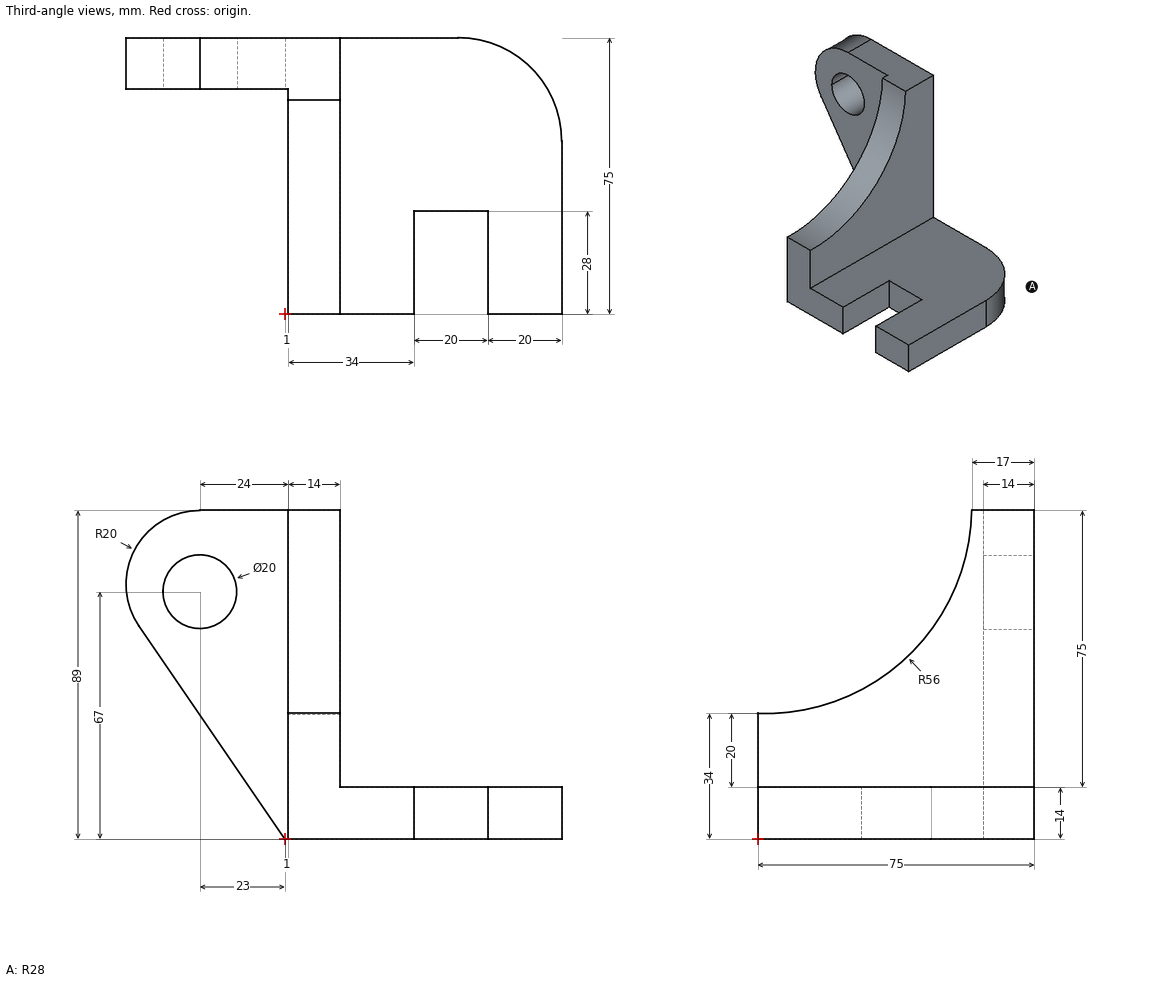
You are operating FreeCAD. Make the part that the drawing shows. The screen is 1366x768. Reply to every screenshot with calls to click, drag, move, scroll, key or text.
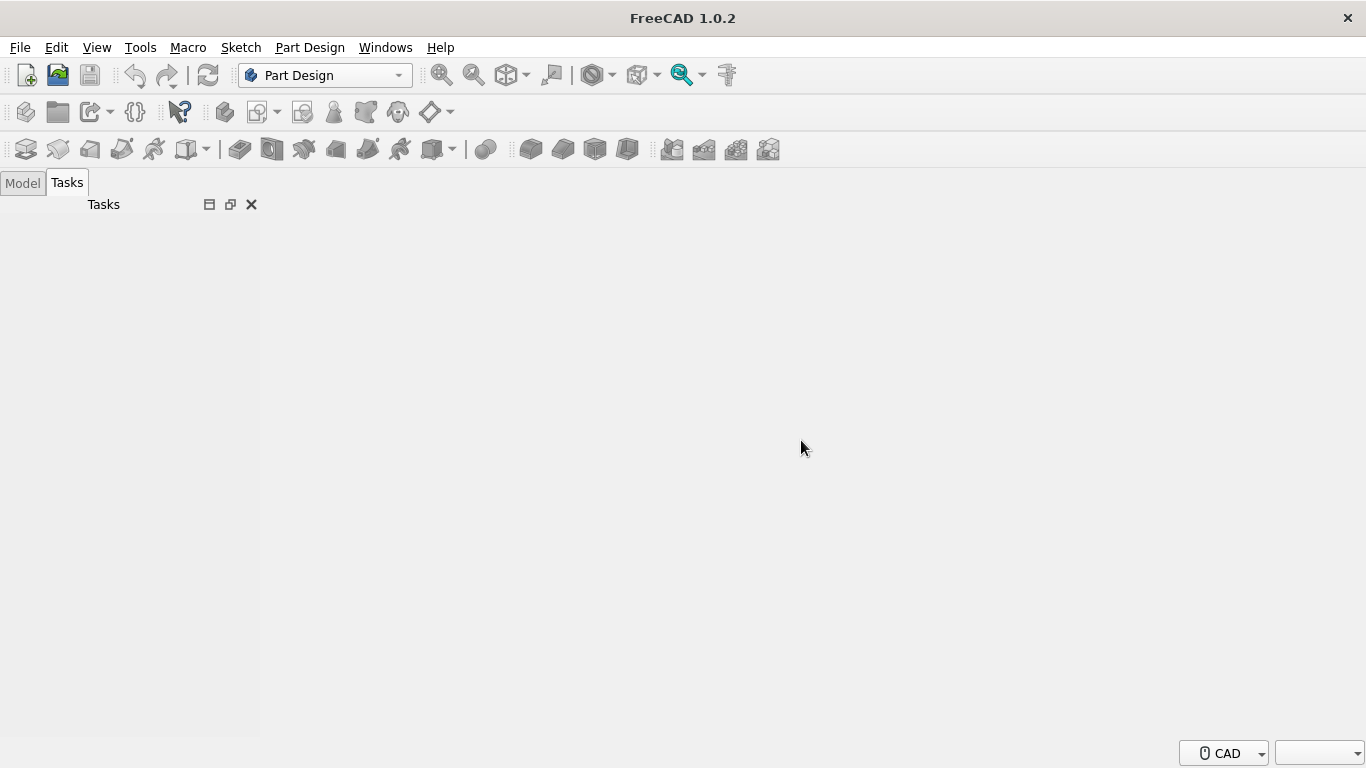
click(26, 76)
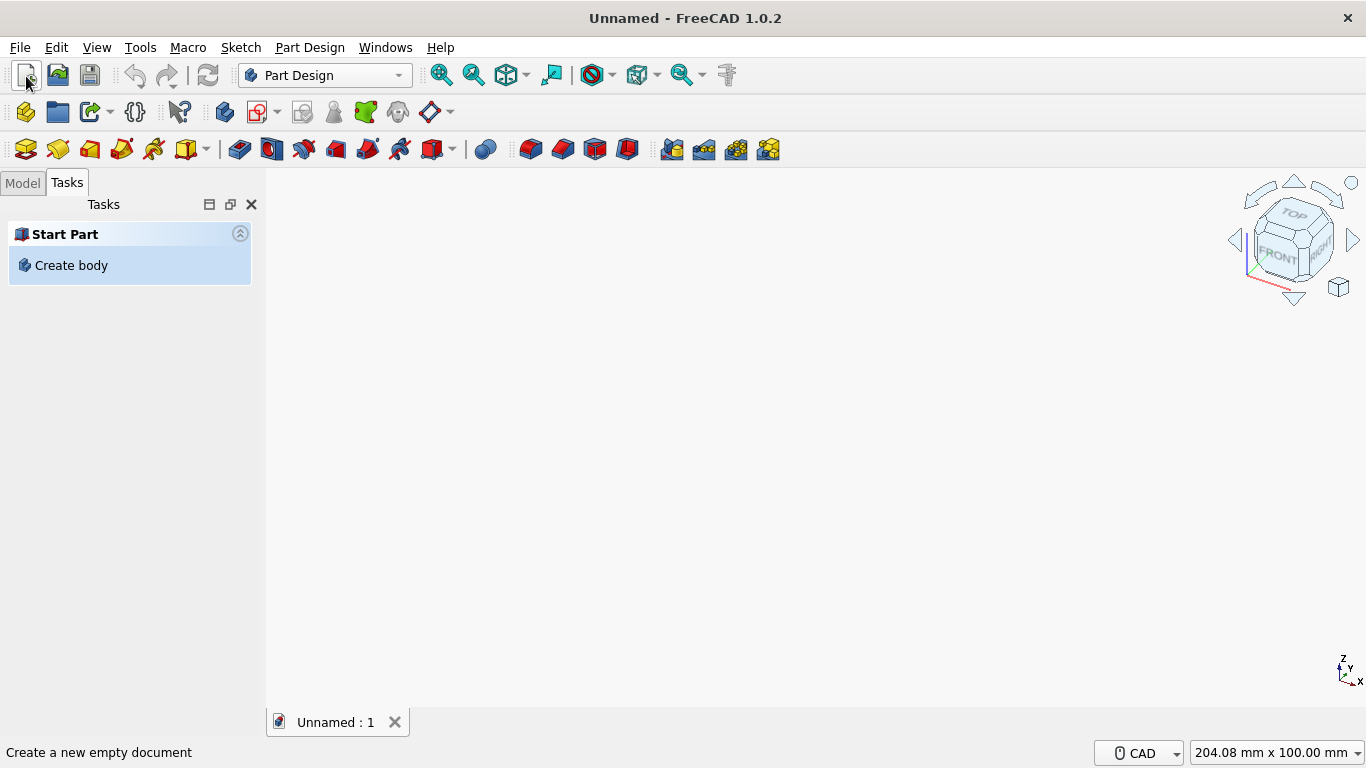
click(258, 112)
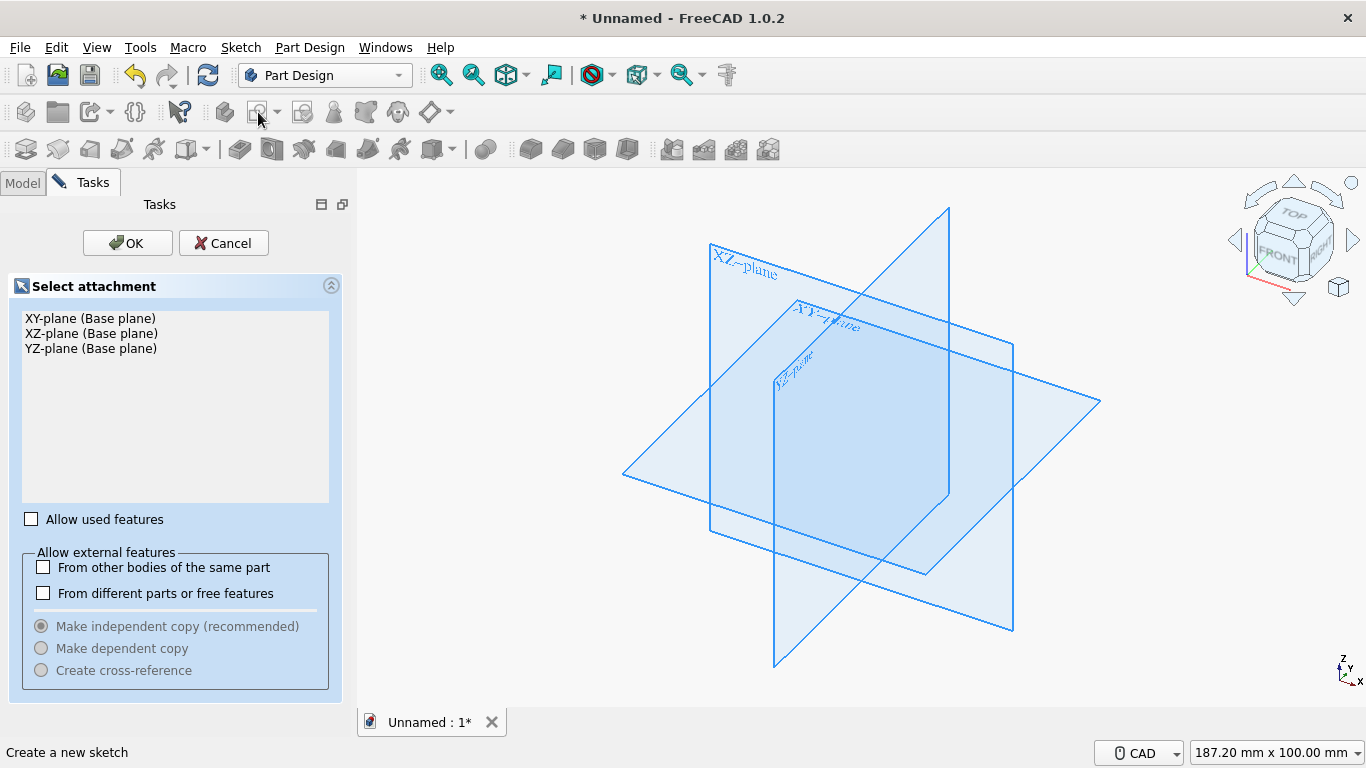
click(82, 318)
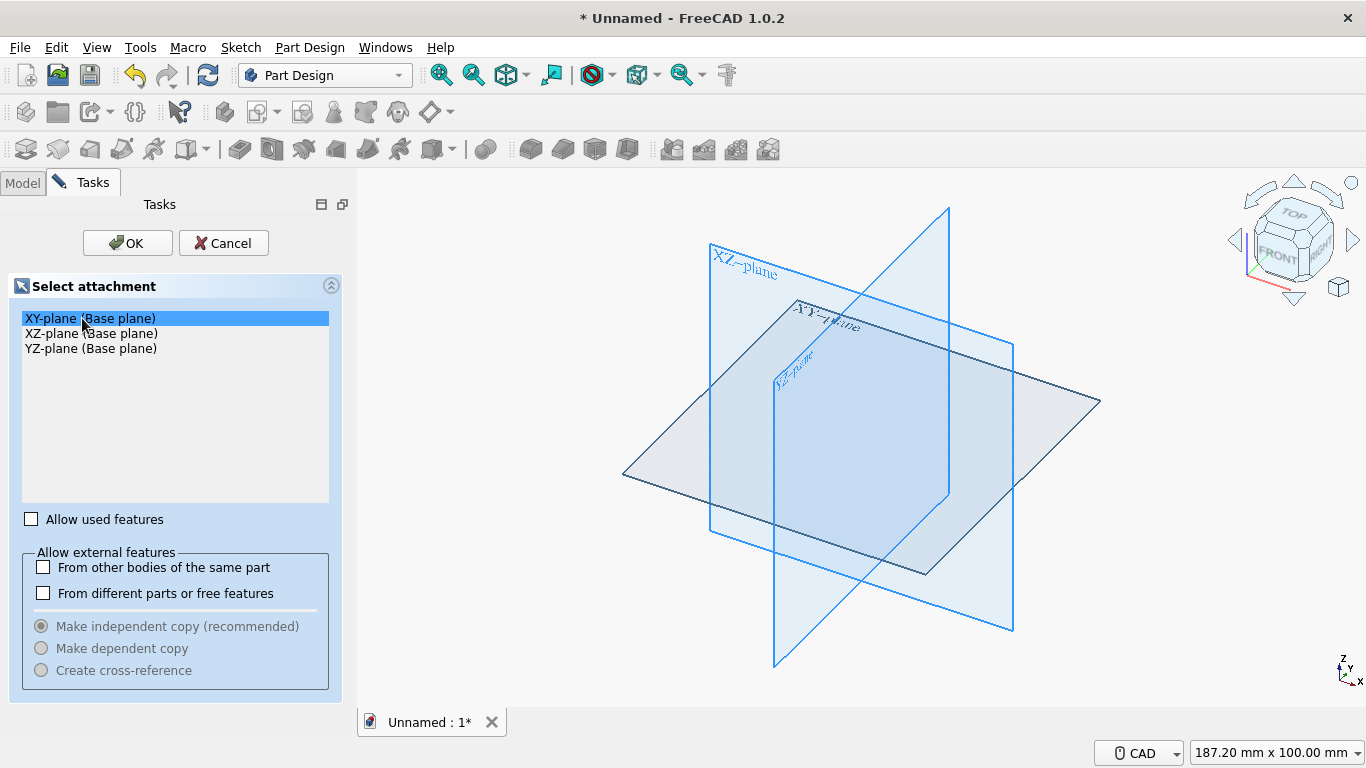
click(128, 243)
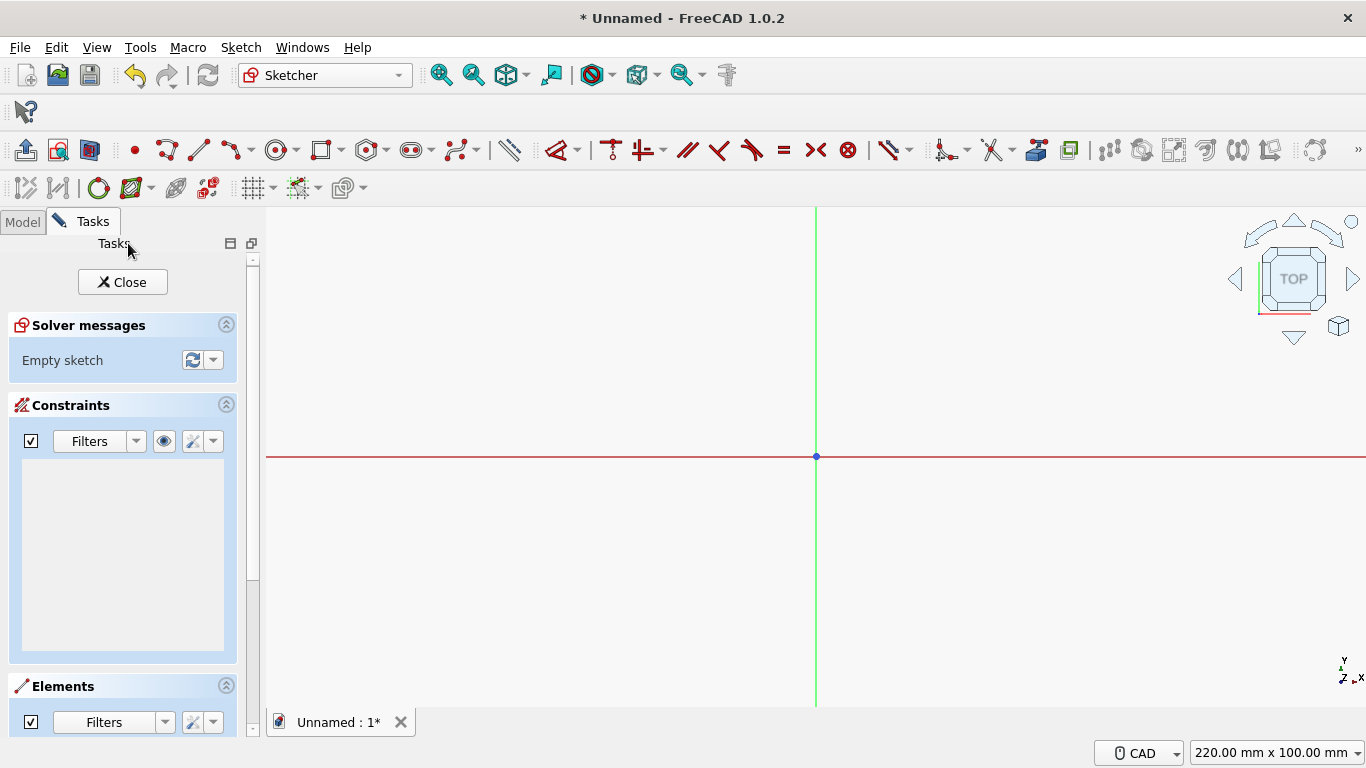
scroll(294, 679, down, 2)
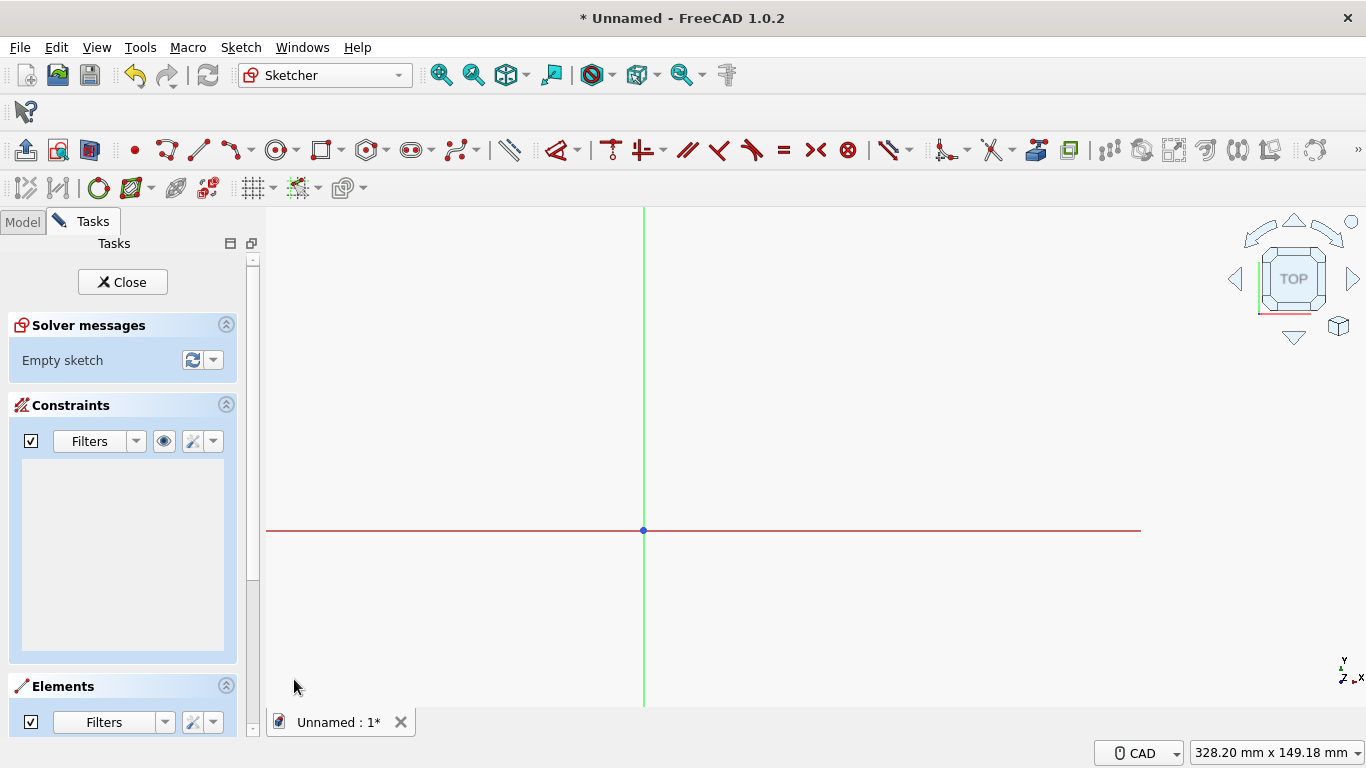
click(168, 150)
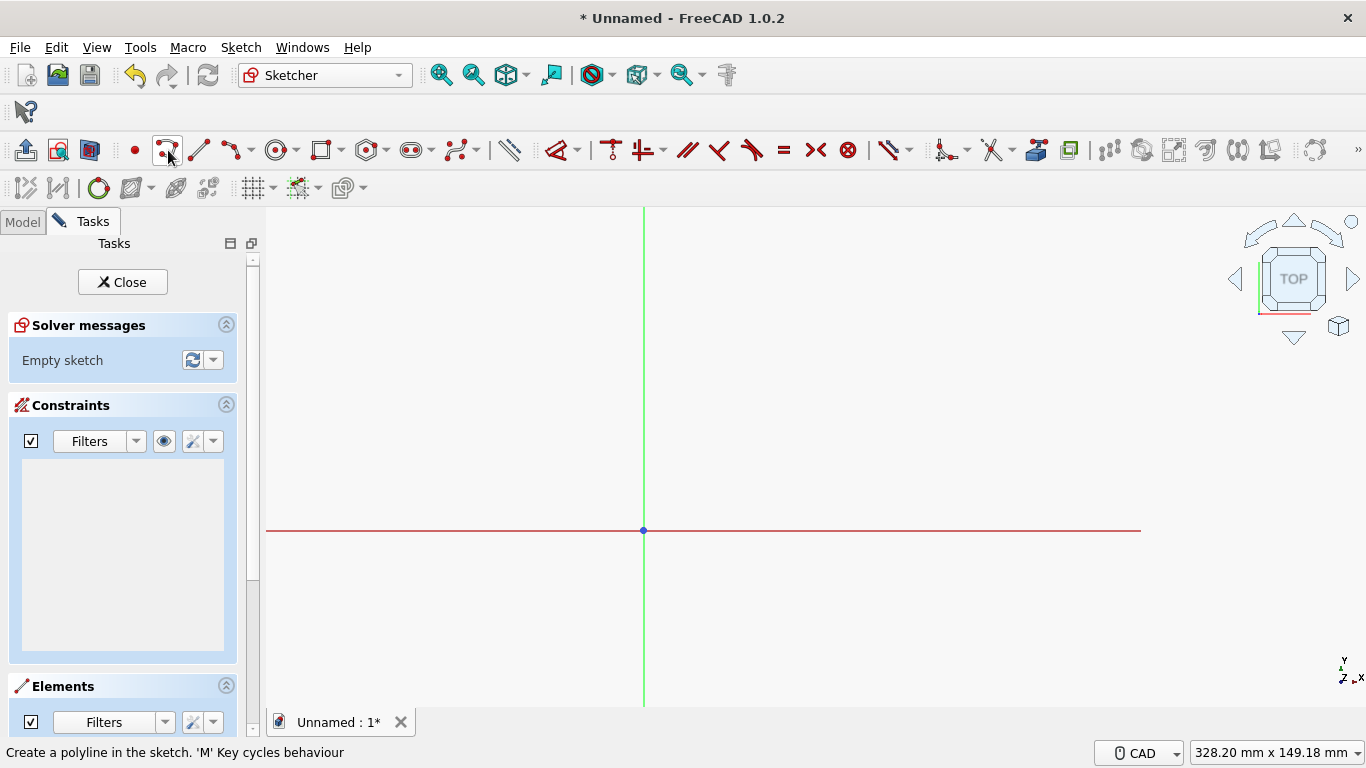
scroll(647, 531, up, 8)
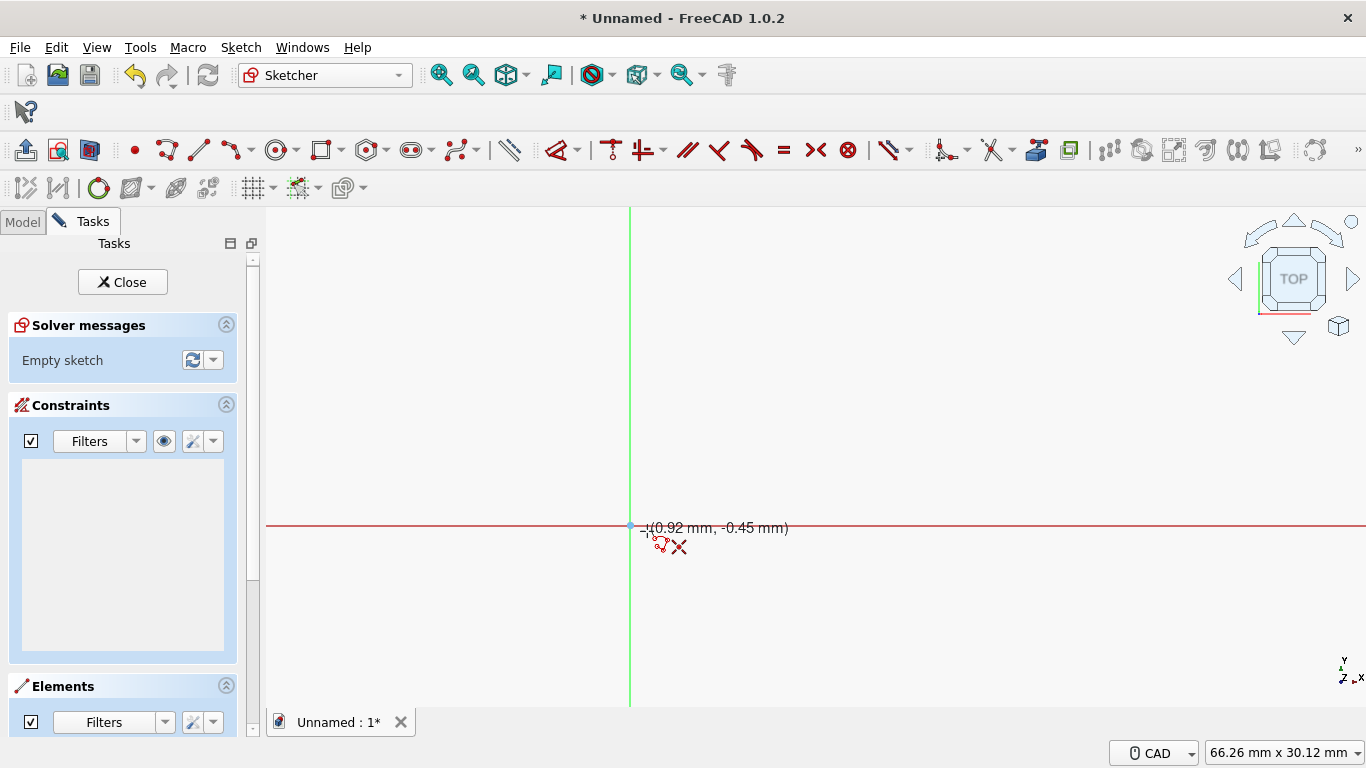
click(647, 526)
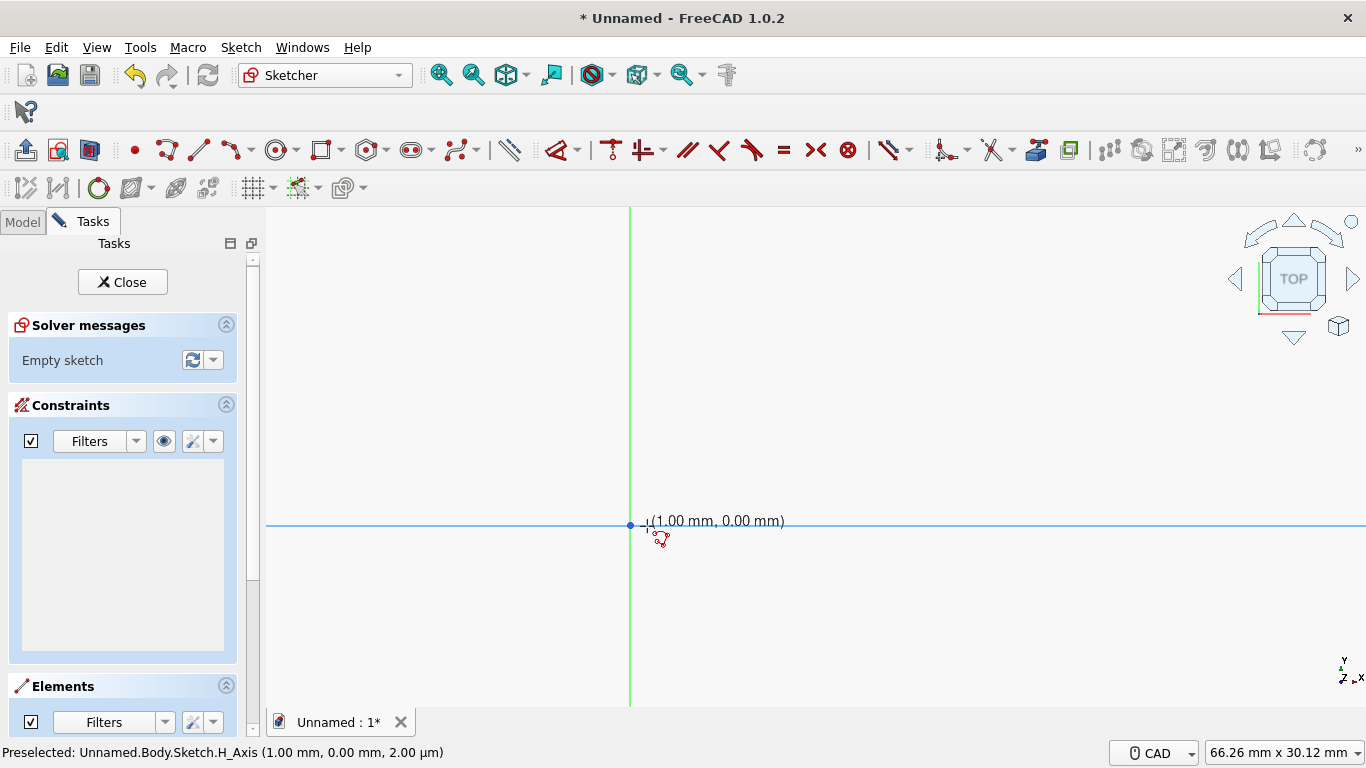
scroll(582, 638, down, 7)